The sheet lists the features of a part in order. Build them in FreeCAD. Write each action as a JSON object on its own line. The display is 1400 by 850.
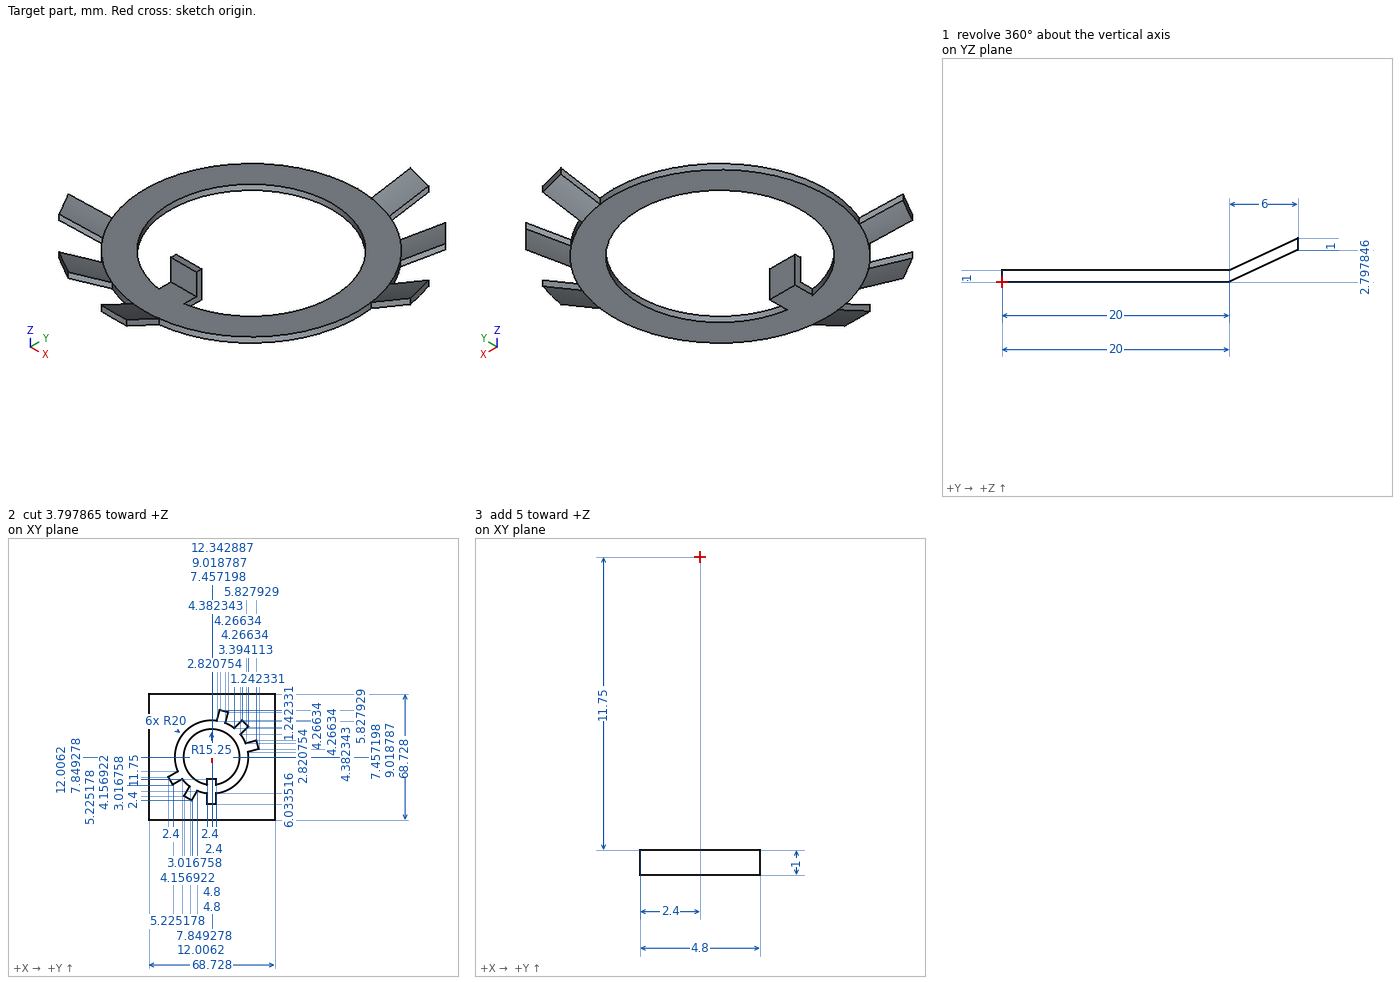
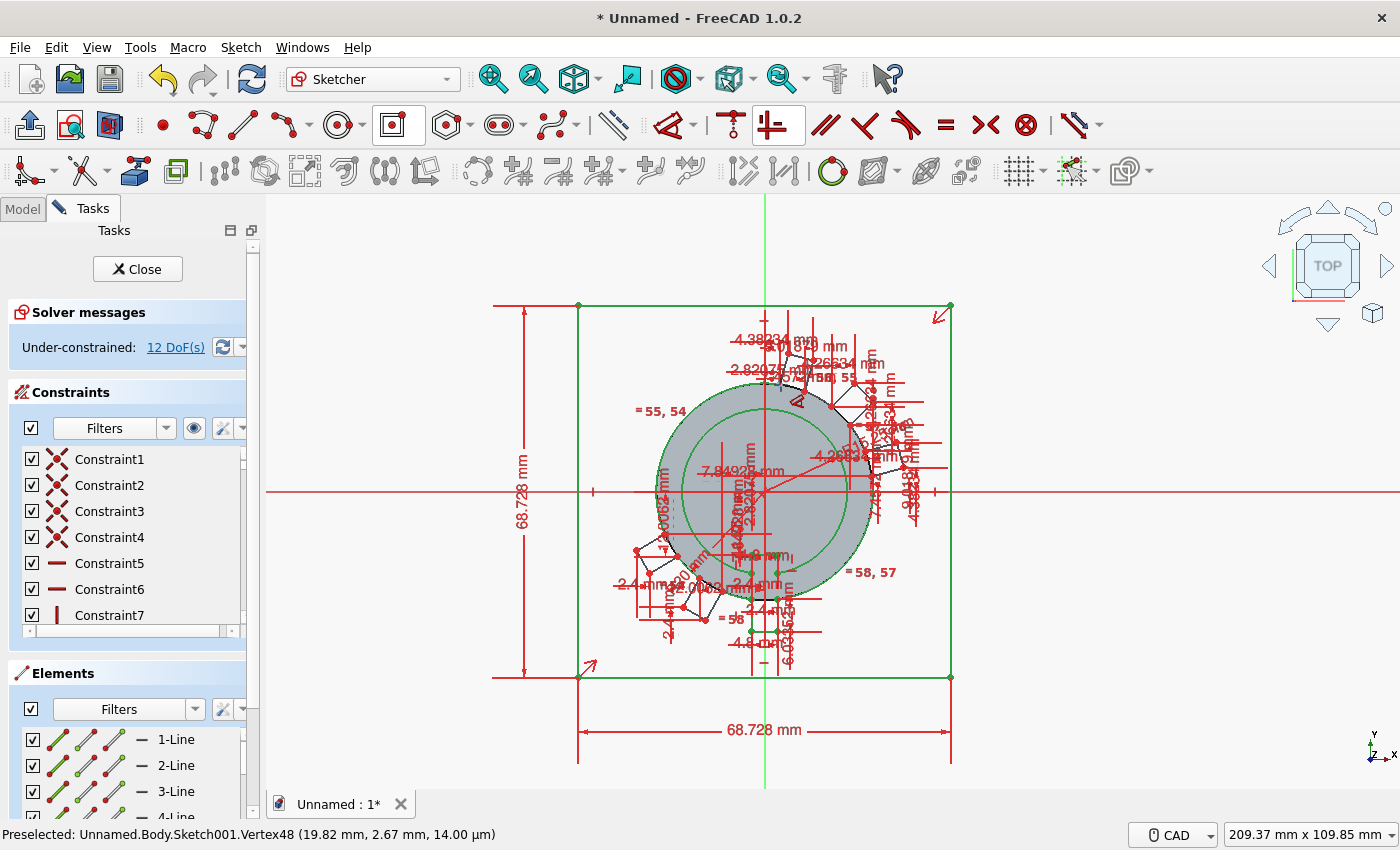
{"action": "scroll", "coordinate": [717, 600], "scroll_direction": "up", "scroll_amount": 5}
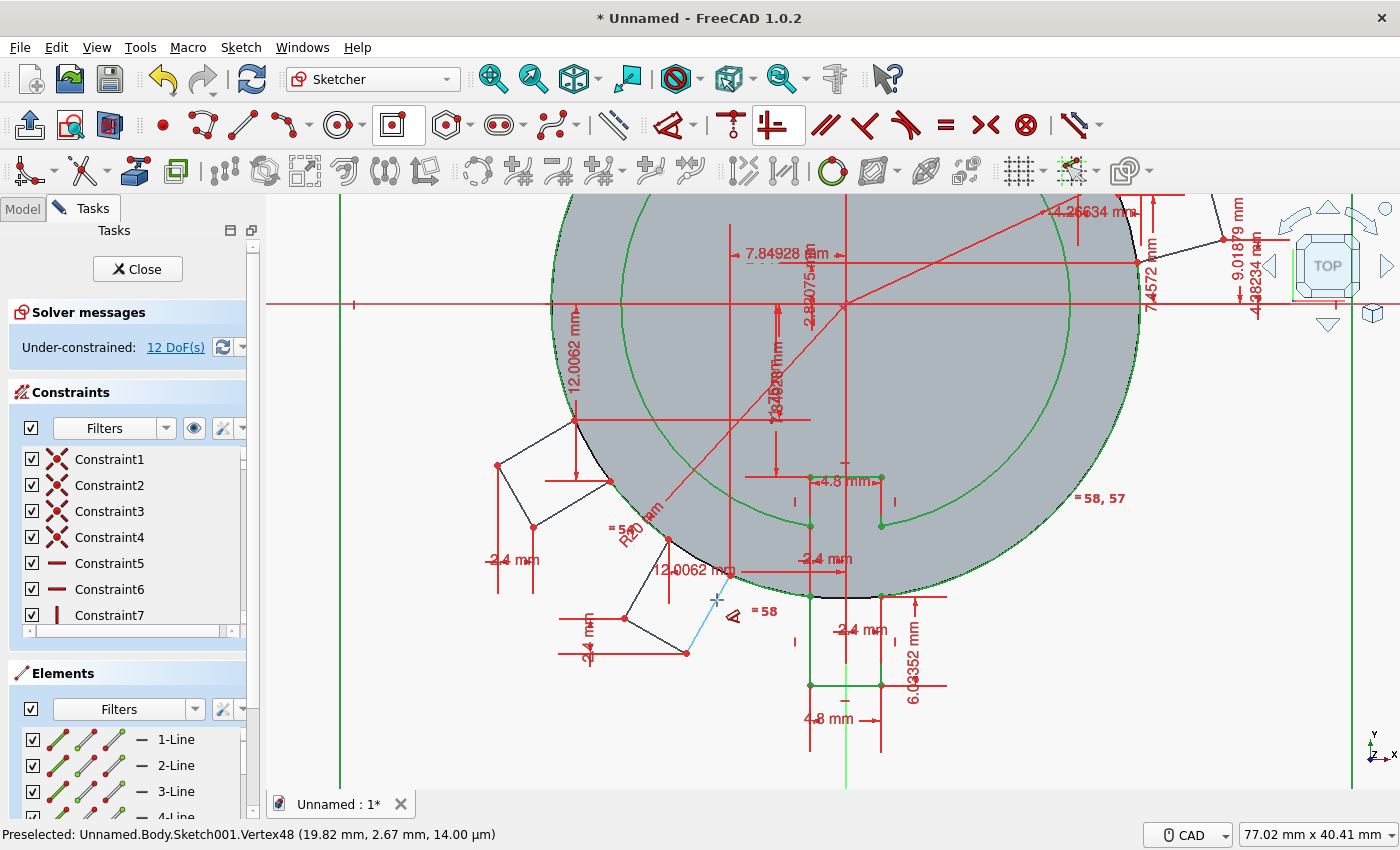
{"action": "left_click", "coordinate": [717, 599]}
{"action": "left_click", "coordinate": [708, 688]}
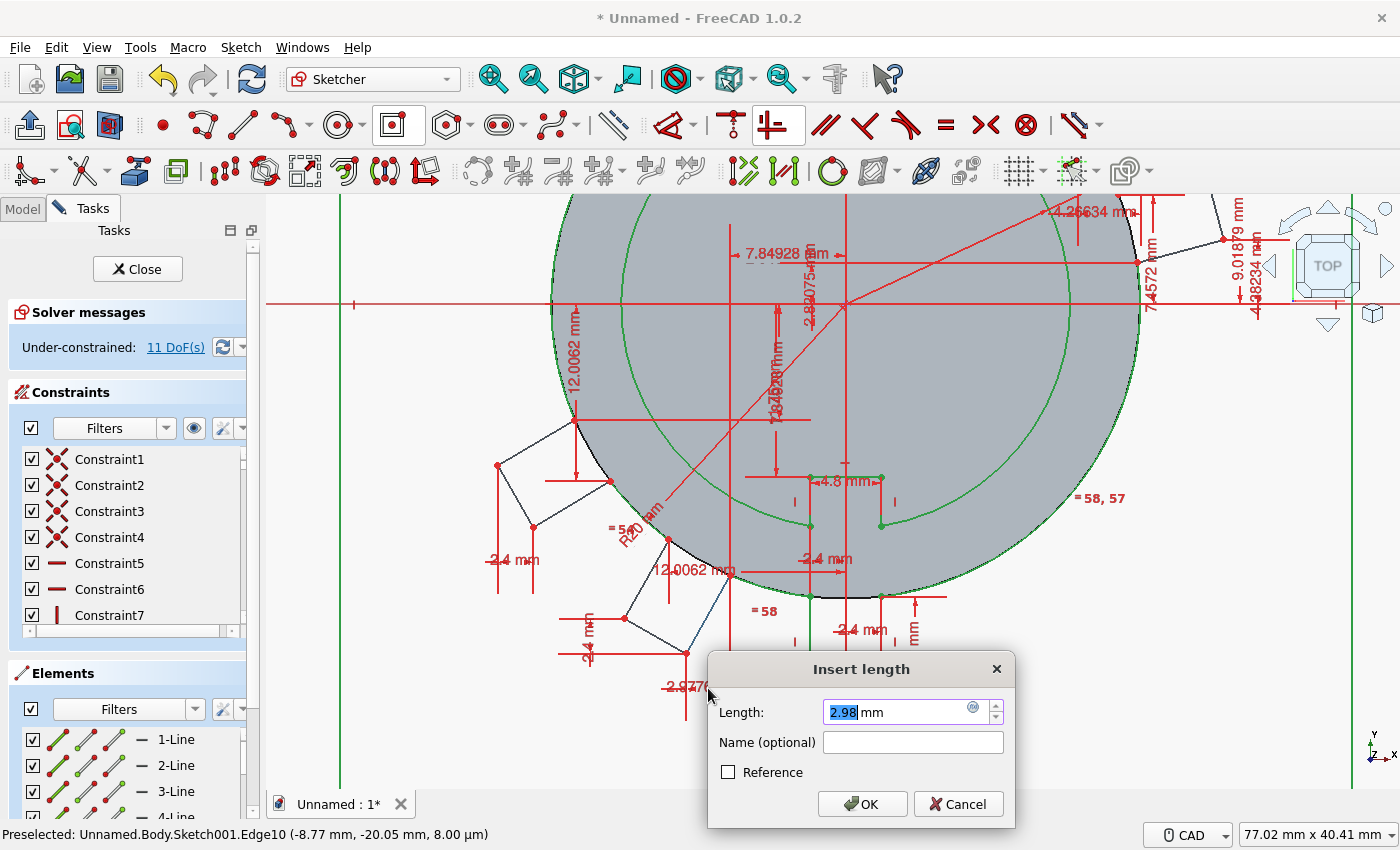
{"action": "type", "text": "3.016758"}
{"action": "key", "text": "Return"}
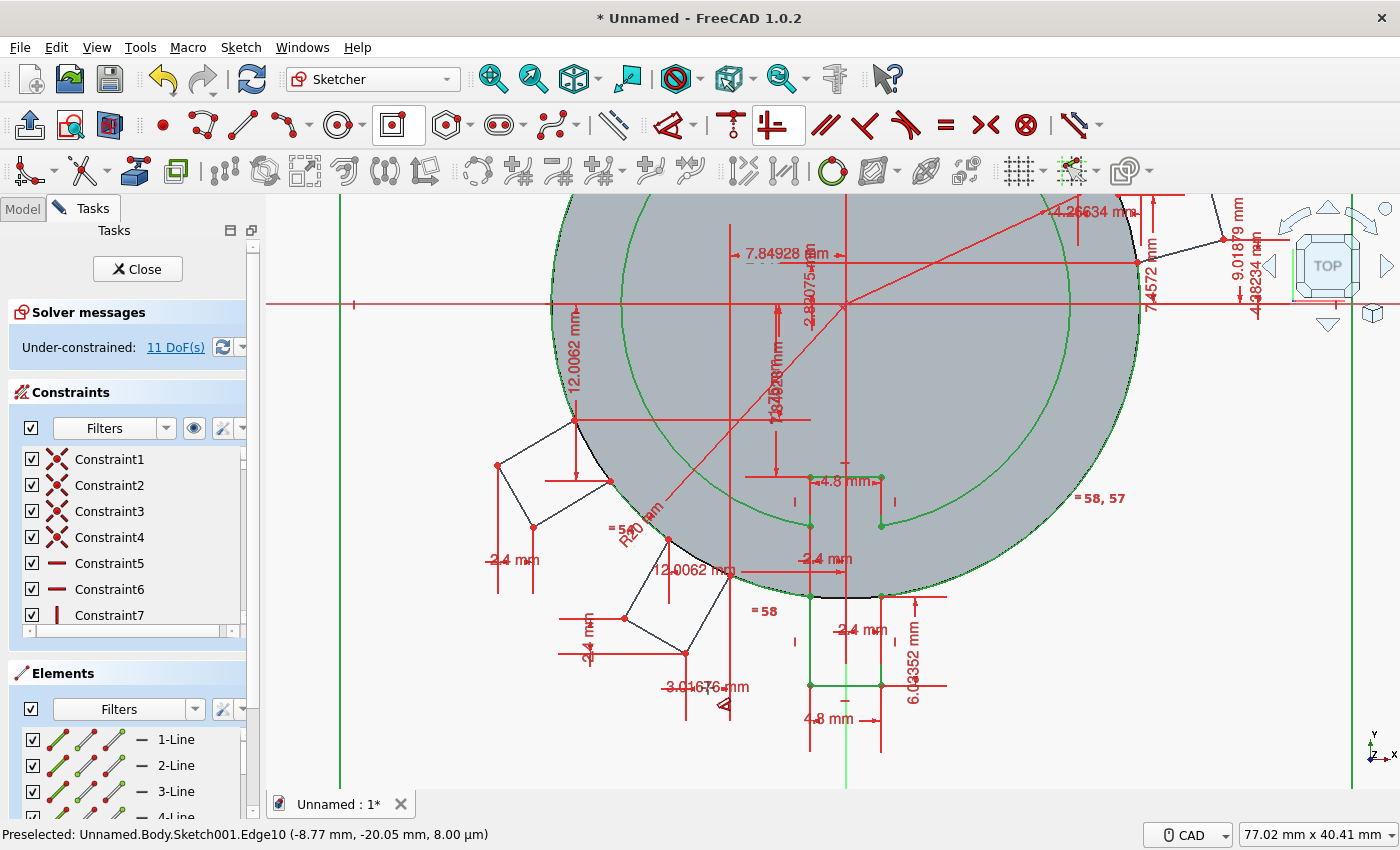
{"action": "left_click", "coordinate": [717, 599]}
{"action": "left_click", "coordinate": [652, 615]}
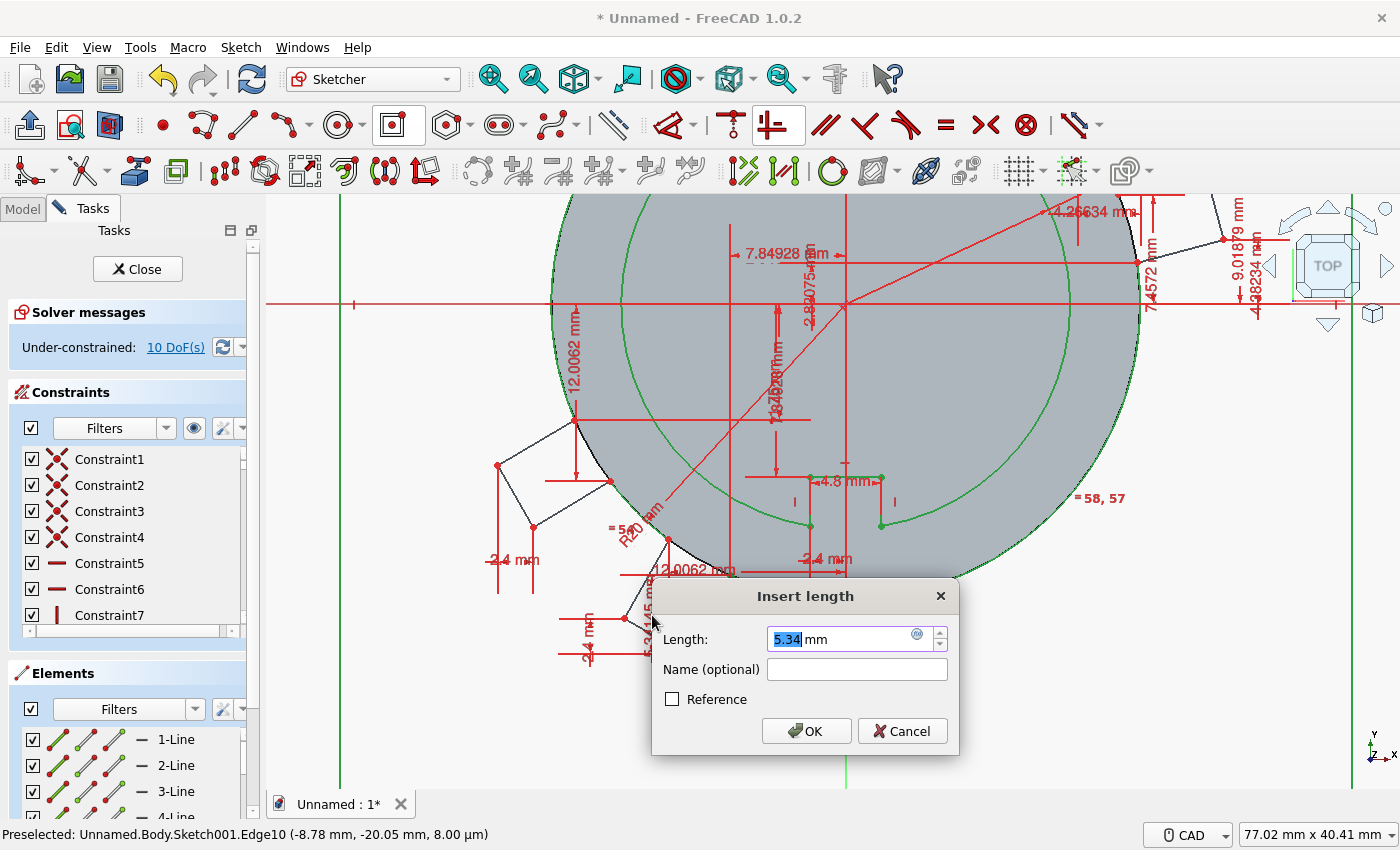
{"action": "type", "text": "5.225178"}
{"action": "key", "text": "Return"}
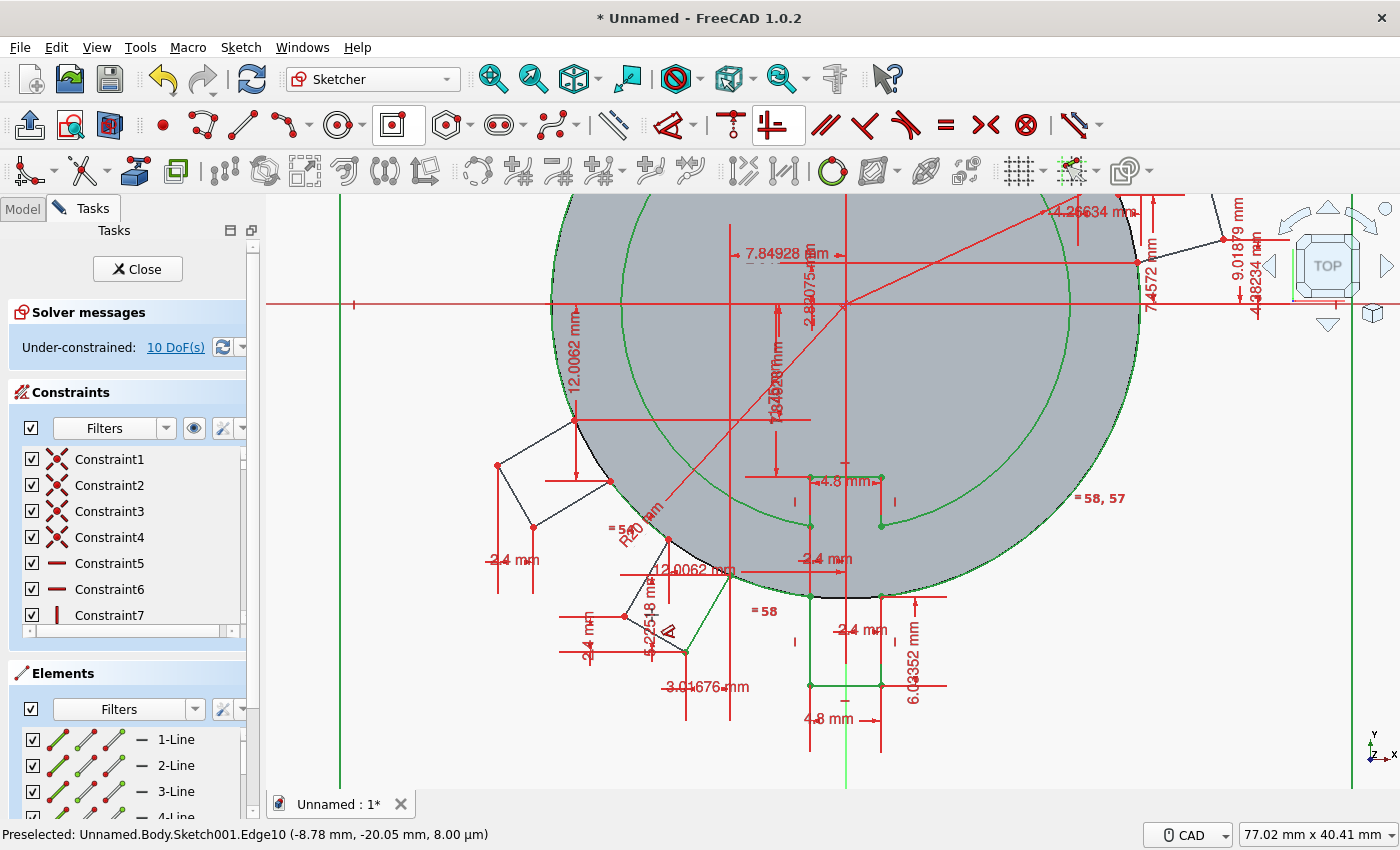
{"action": "left_click", "coordinate": [667, 642]}
{"action": "left_click", "coordinate": [634, 686]}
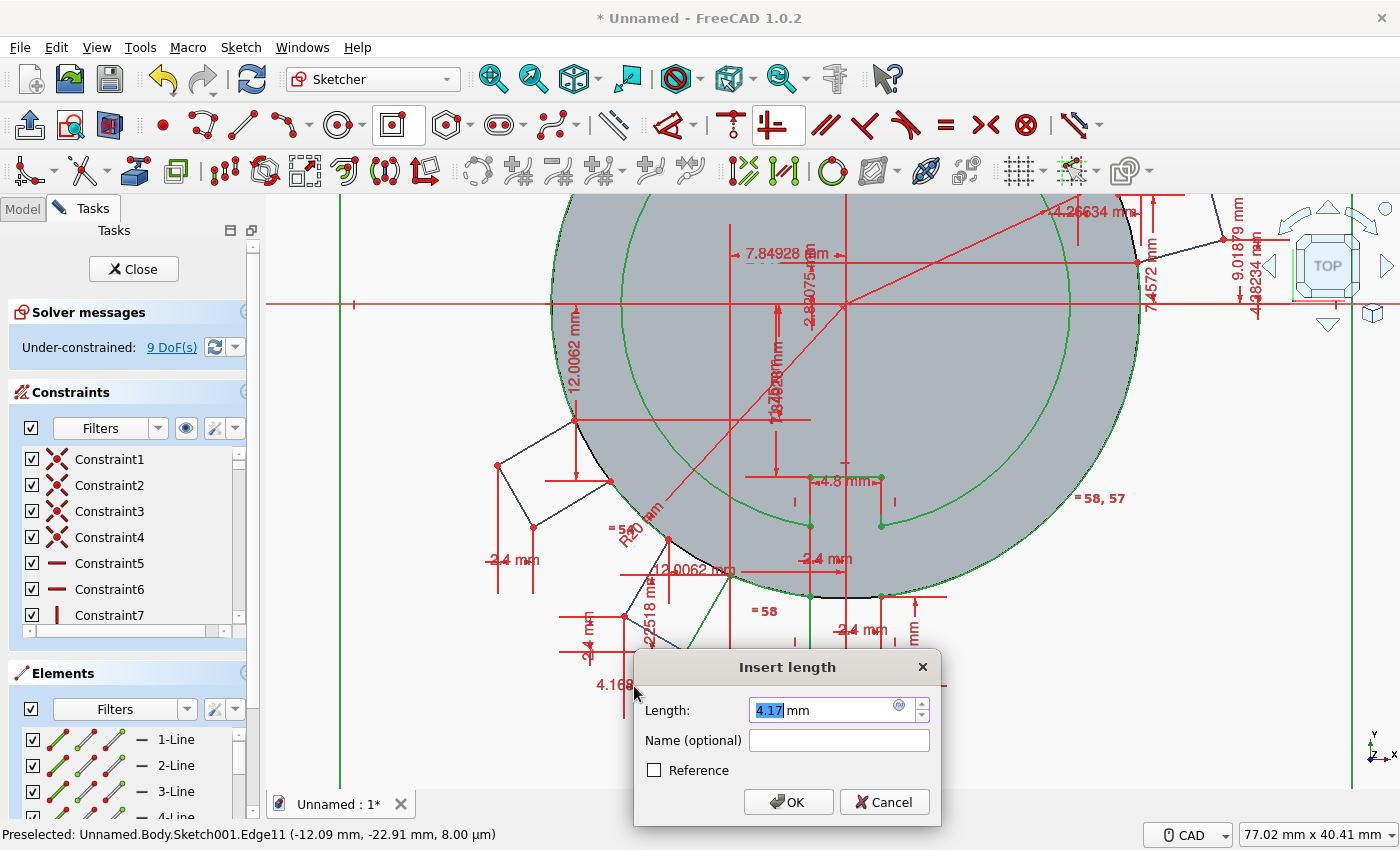
{"action": "type", "text": "4.156922"}
{"action": "key", "text": "Return"}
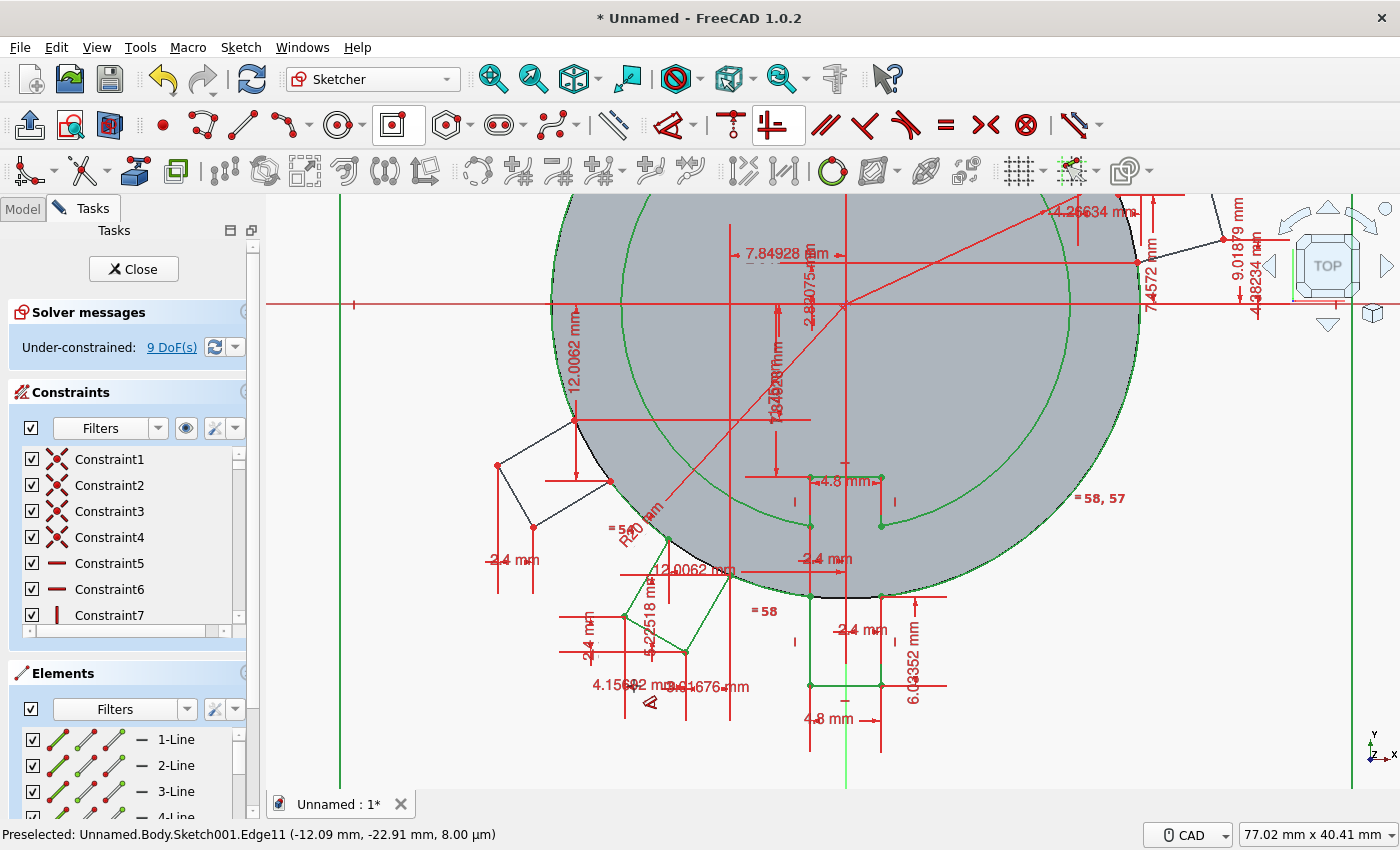
{"action": "left_click", "coordinate": [587, 495]}
{"action": "left_click", "coordinate": [589, 562]}